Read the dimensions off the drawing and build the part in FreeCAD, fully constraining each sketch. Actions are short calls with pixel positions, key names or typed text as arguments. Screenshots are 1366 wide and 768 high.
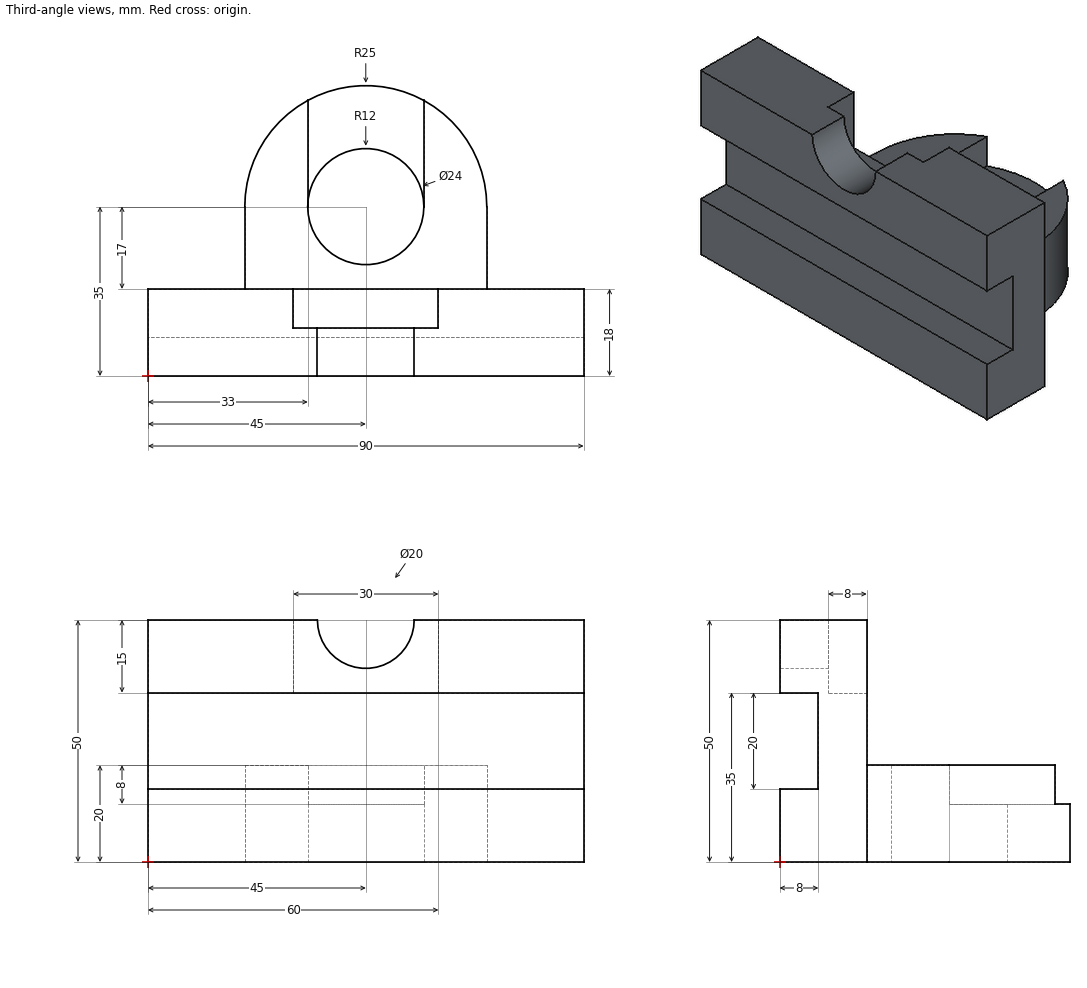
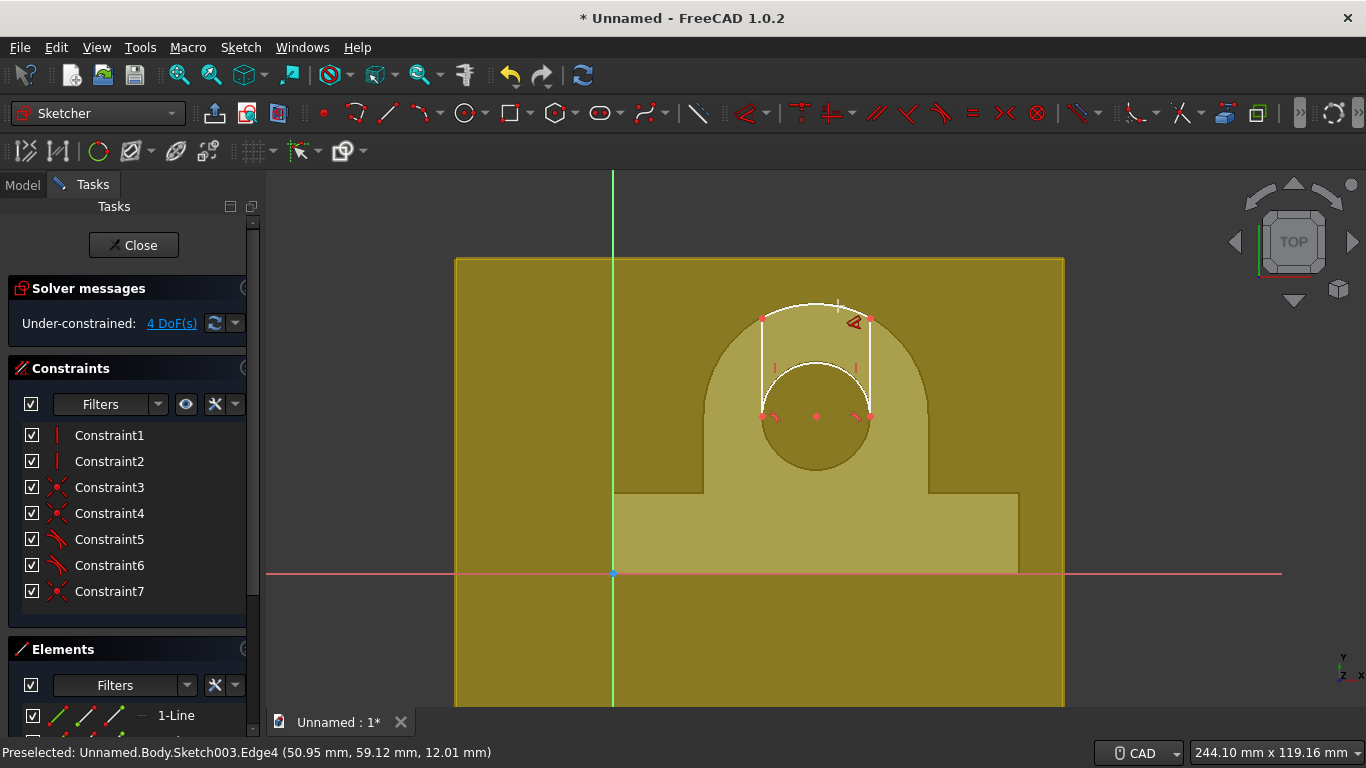
click(848, 373)
click(894, 380)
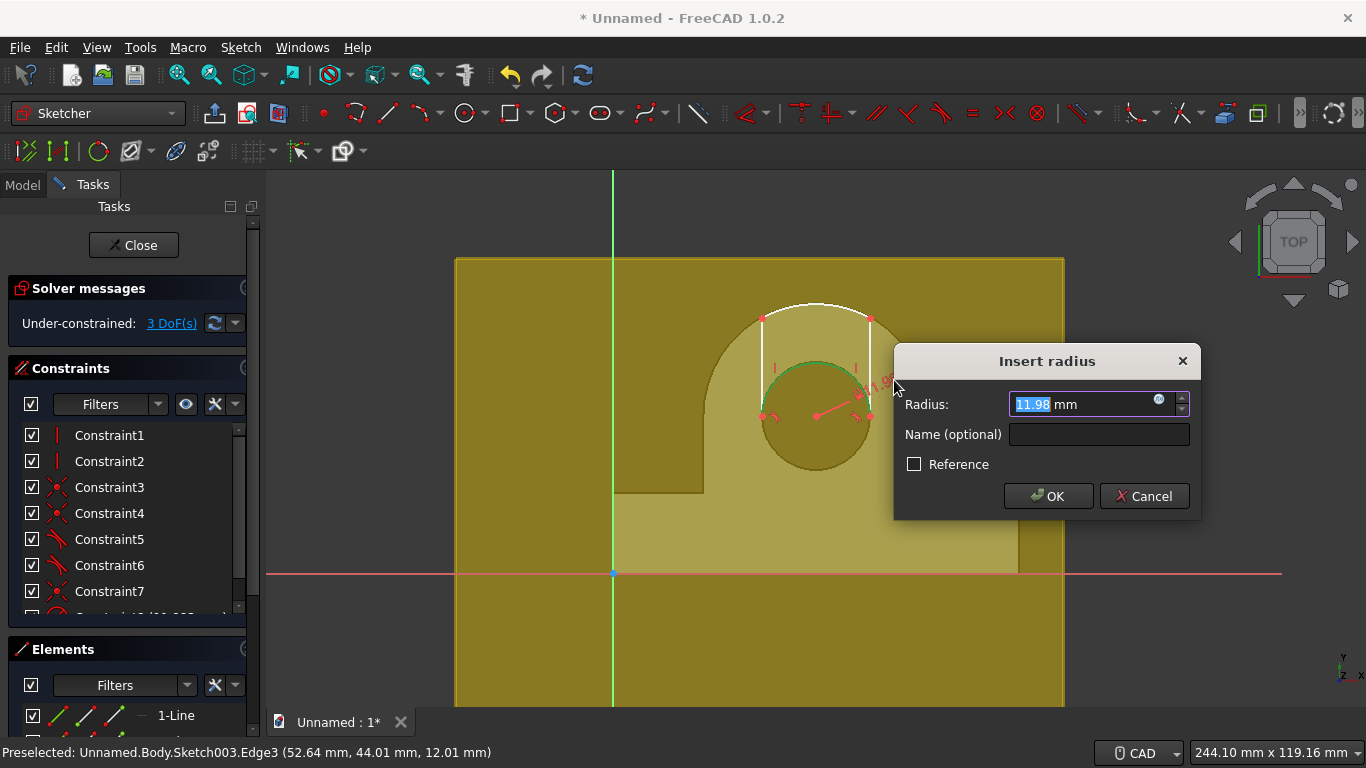
text(12)
key(Return)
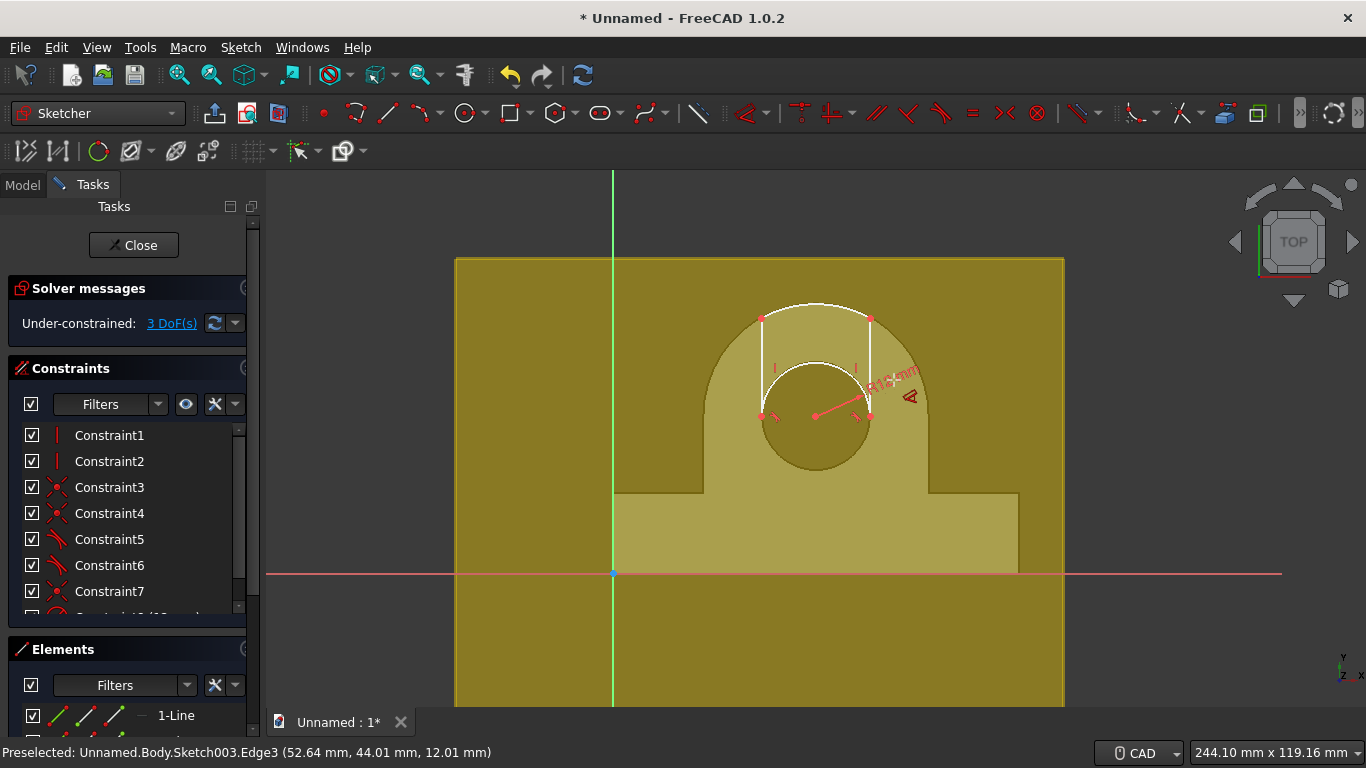
click(838, 306)
click(844, 275)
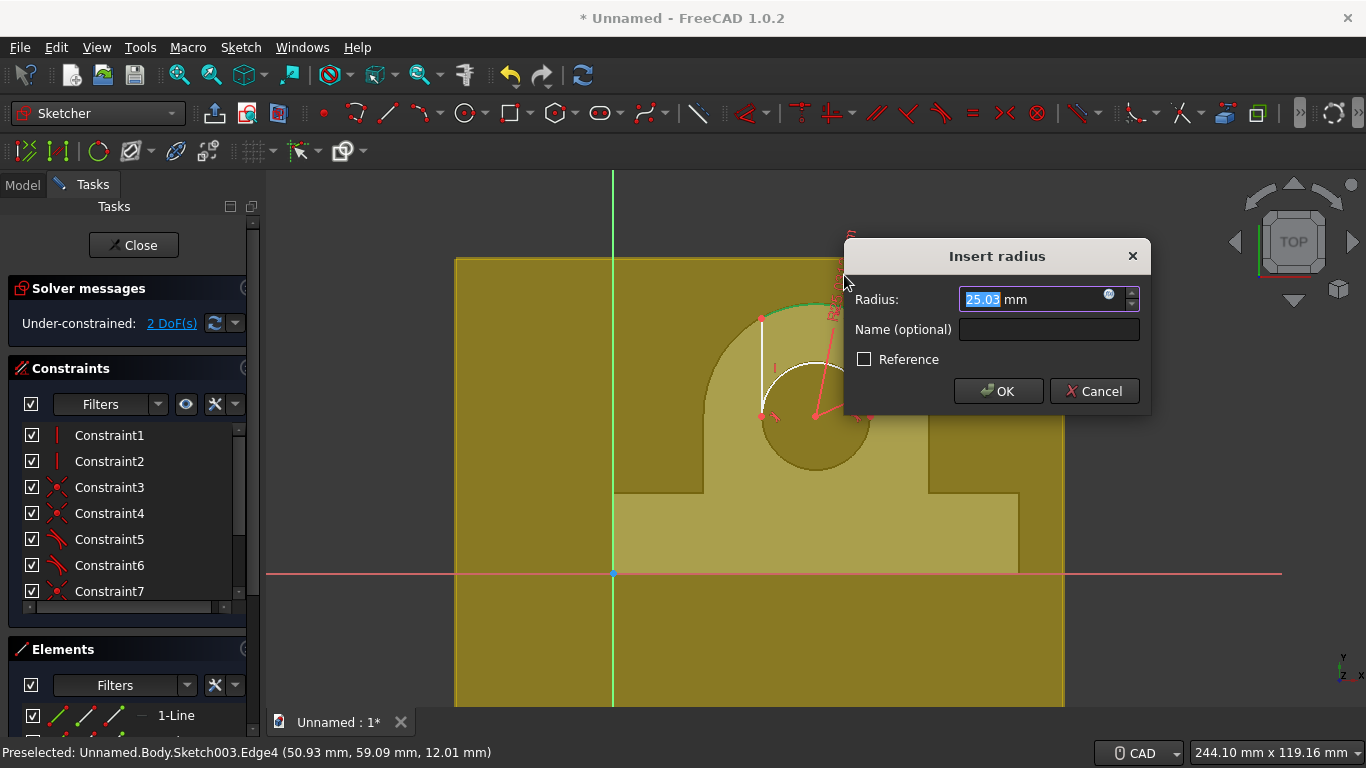
text(25)
key(Return)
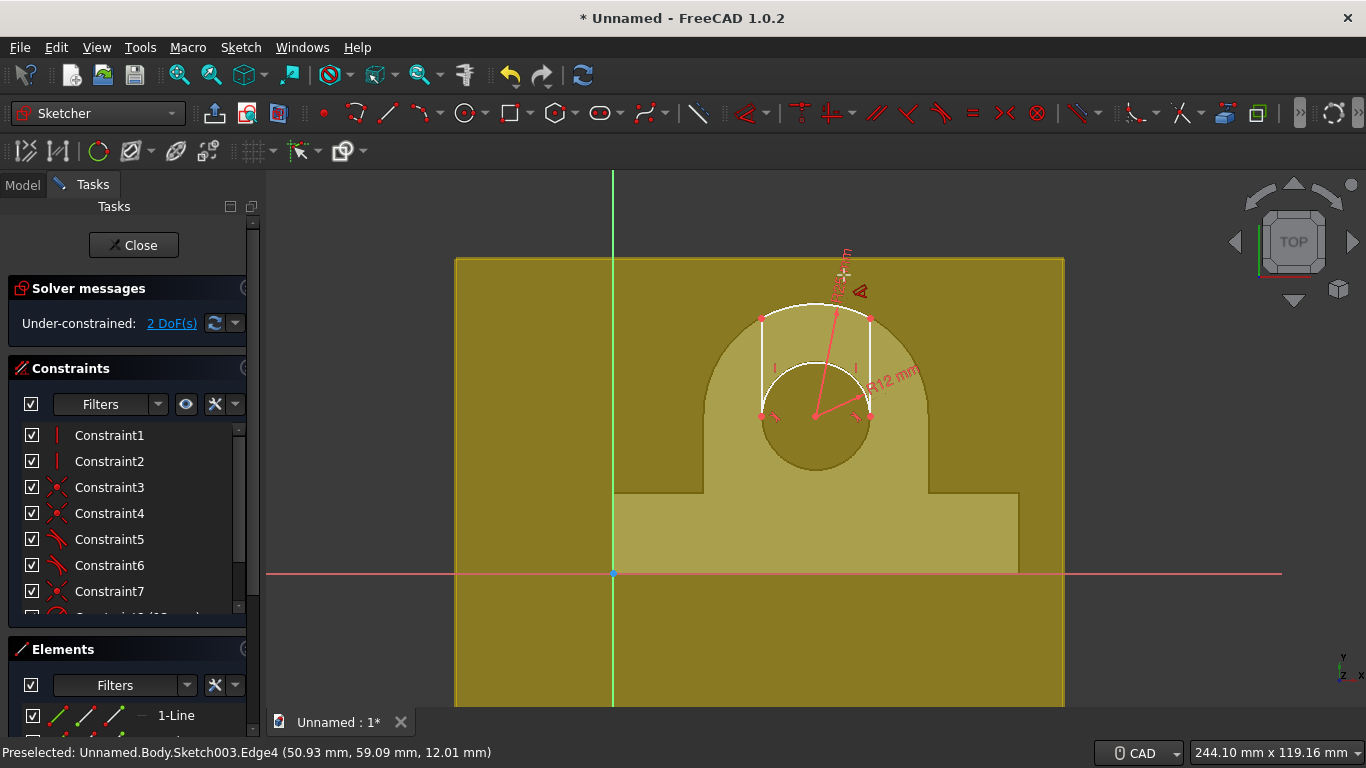
click(762, 318)
click(688, 608)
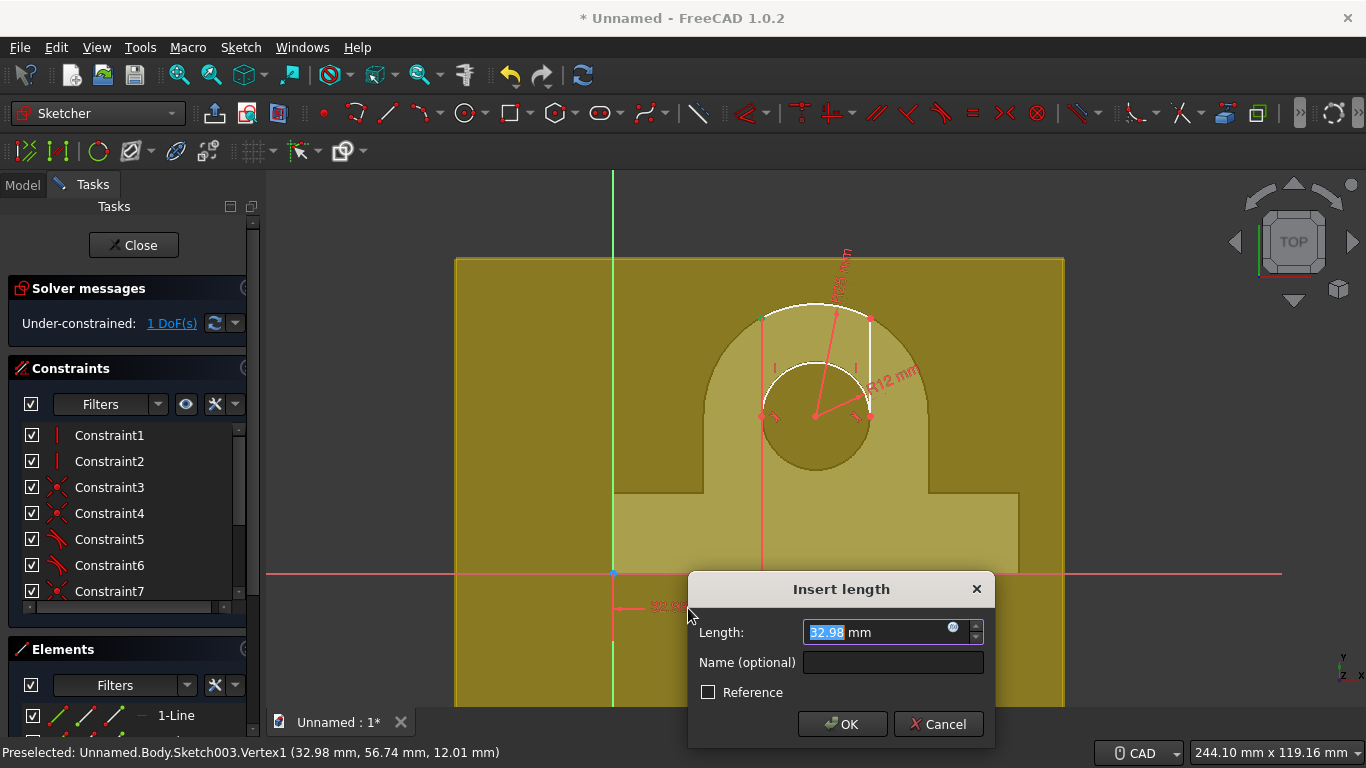
text(33)
key(Return)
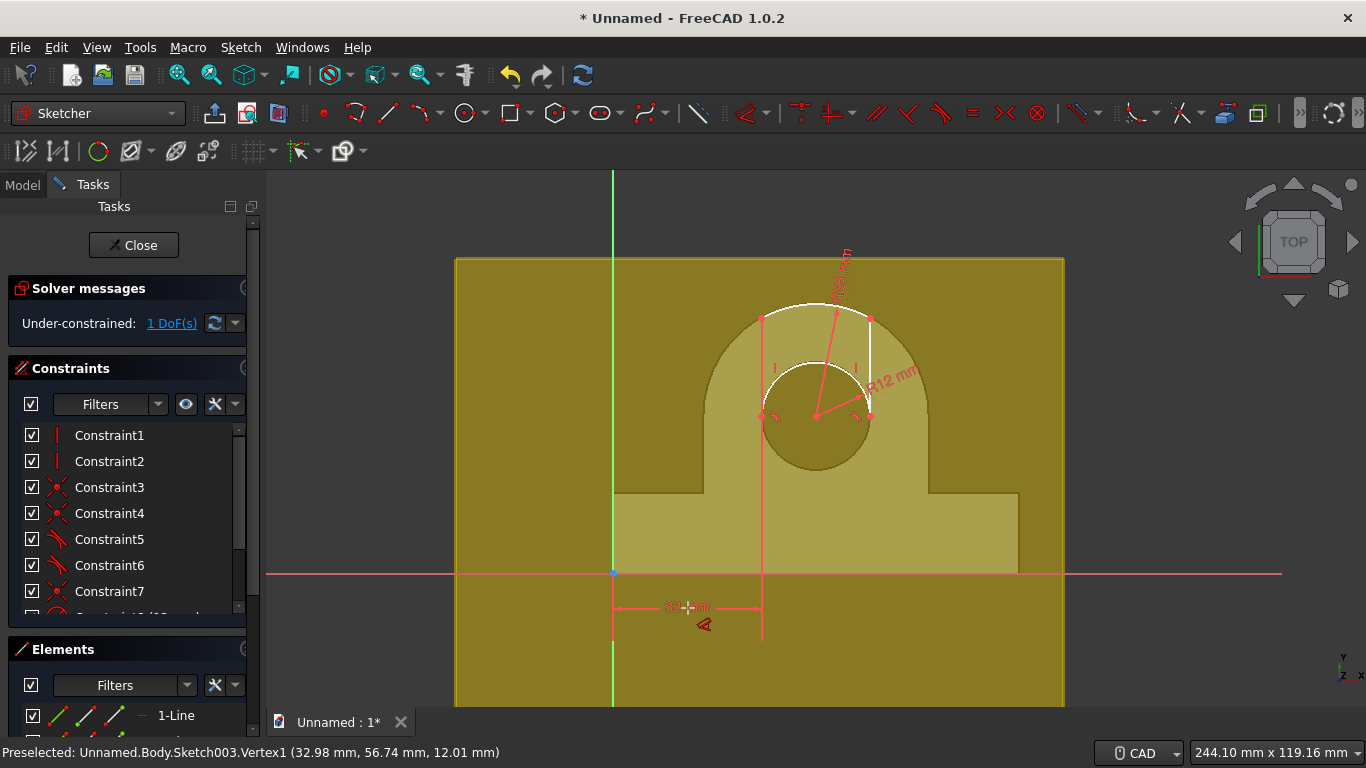
click(762, 417)
click(579, 495)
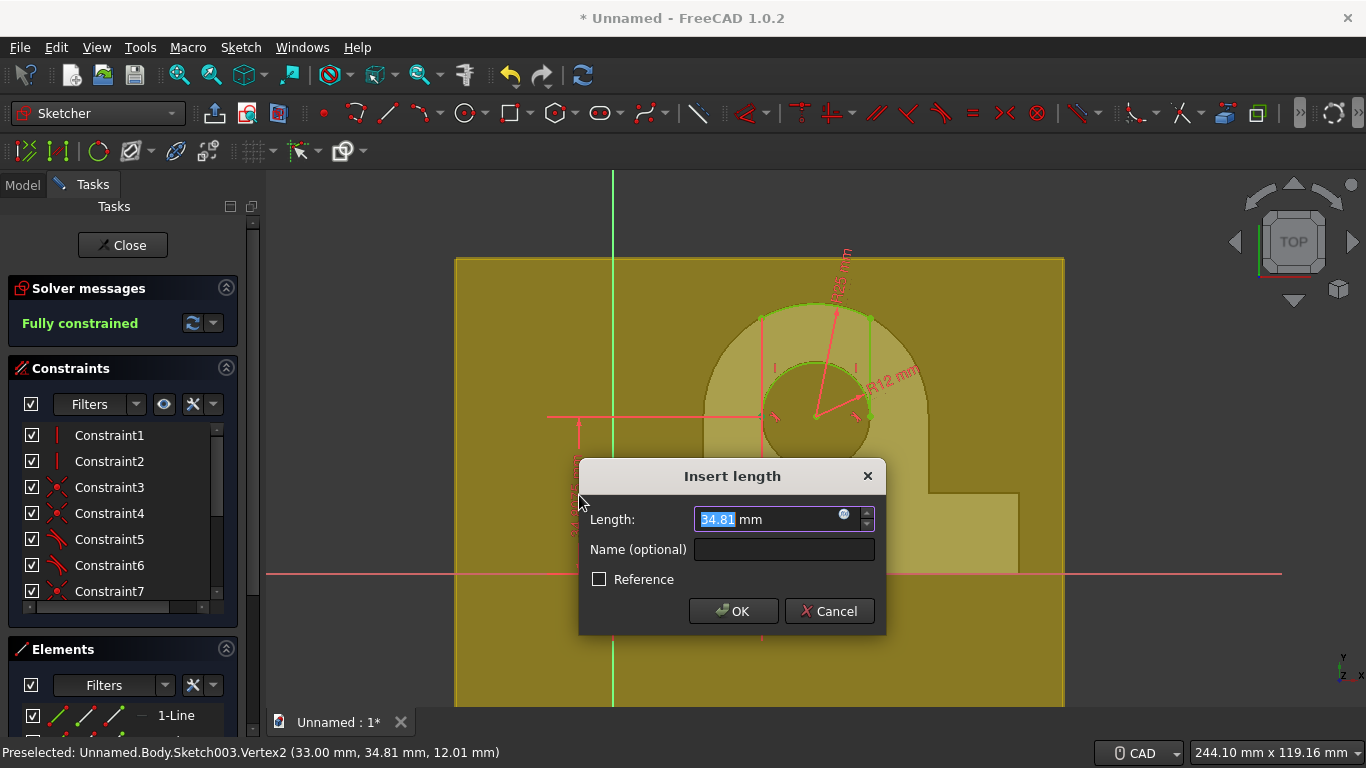
text(35)
key(Return)
key(Escape)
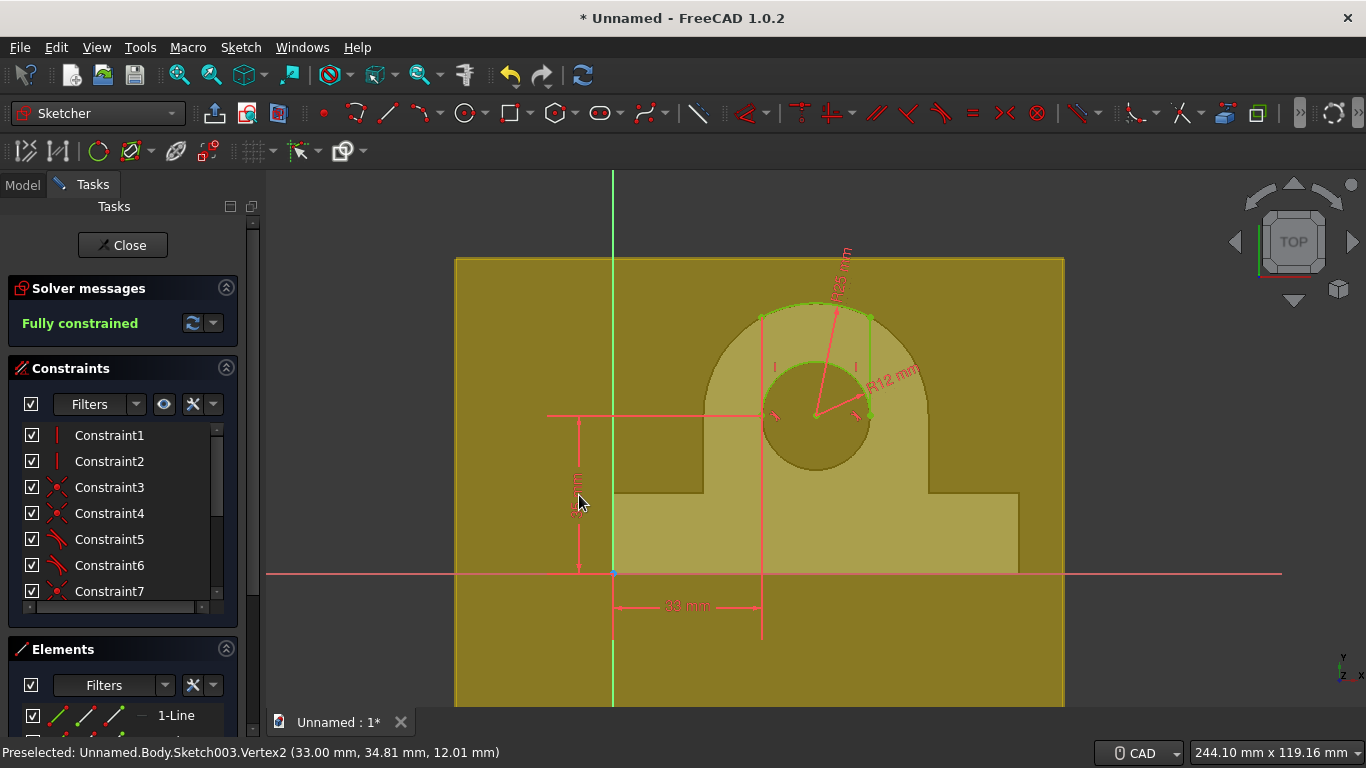
click(123, 245)